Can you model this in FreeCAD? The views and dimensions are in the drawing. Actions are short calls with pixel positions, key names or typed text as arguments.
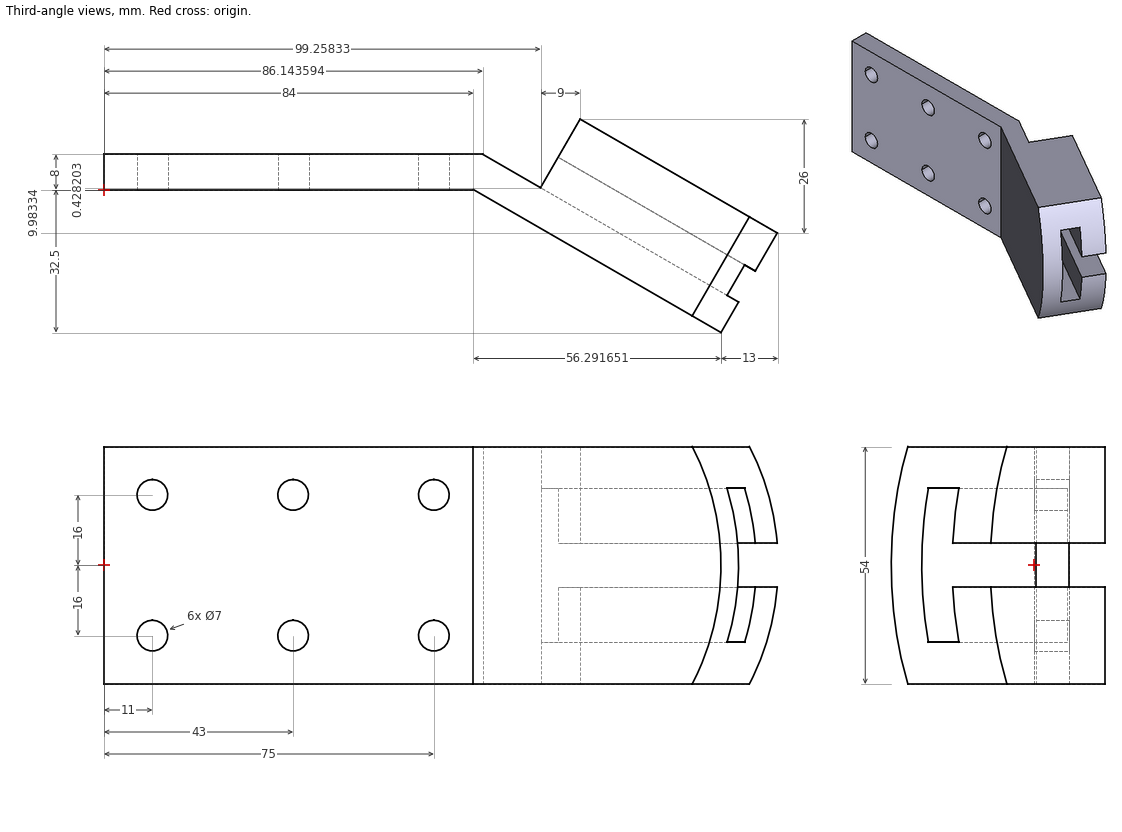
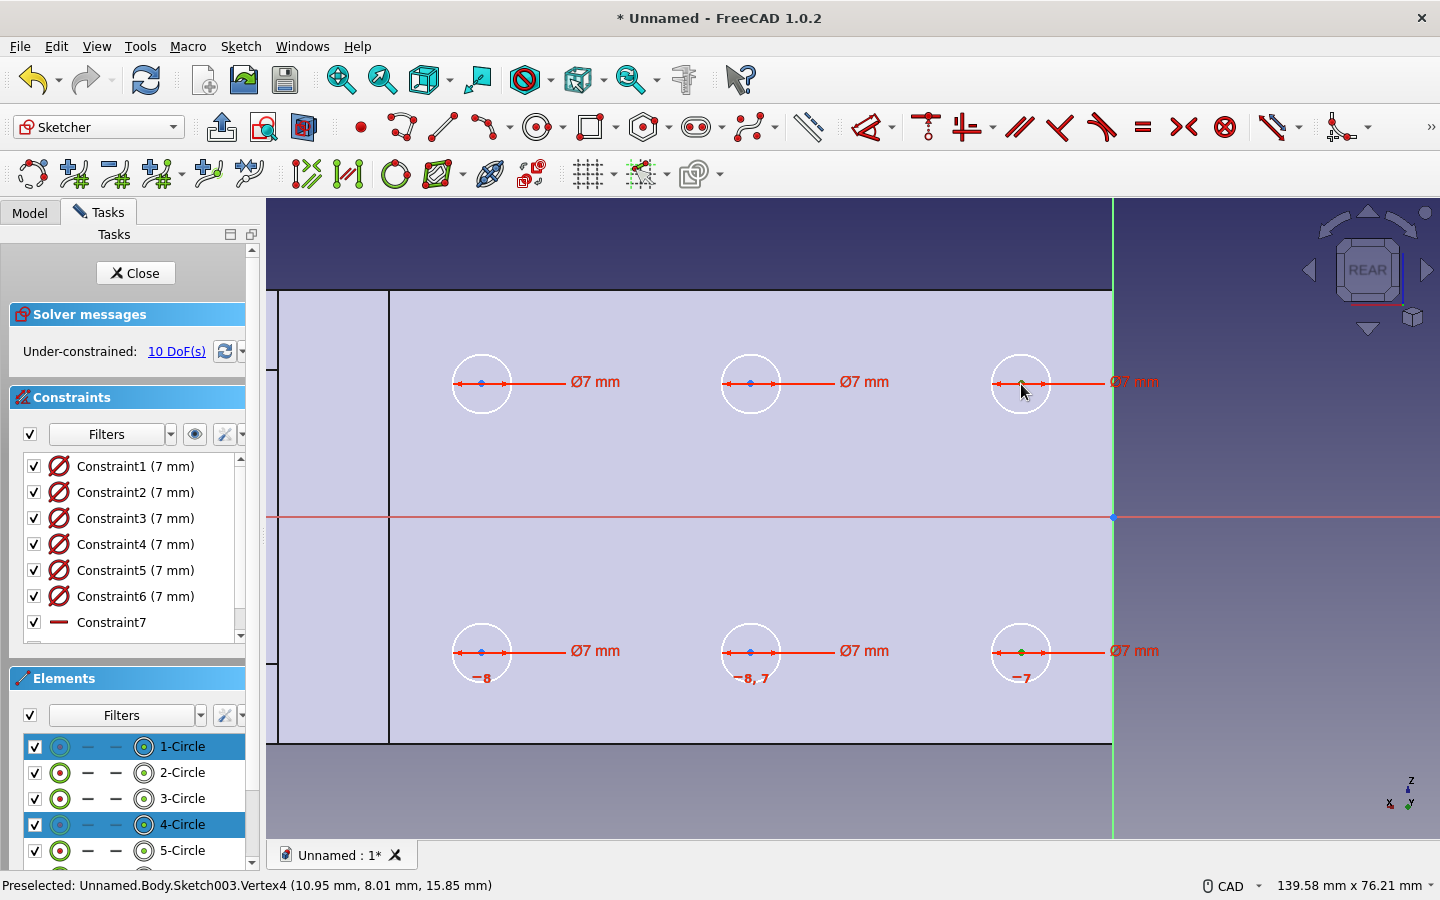
key(v)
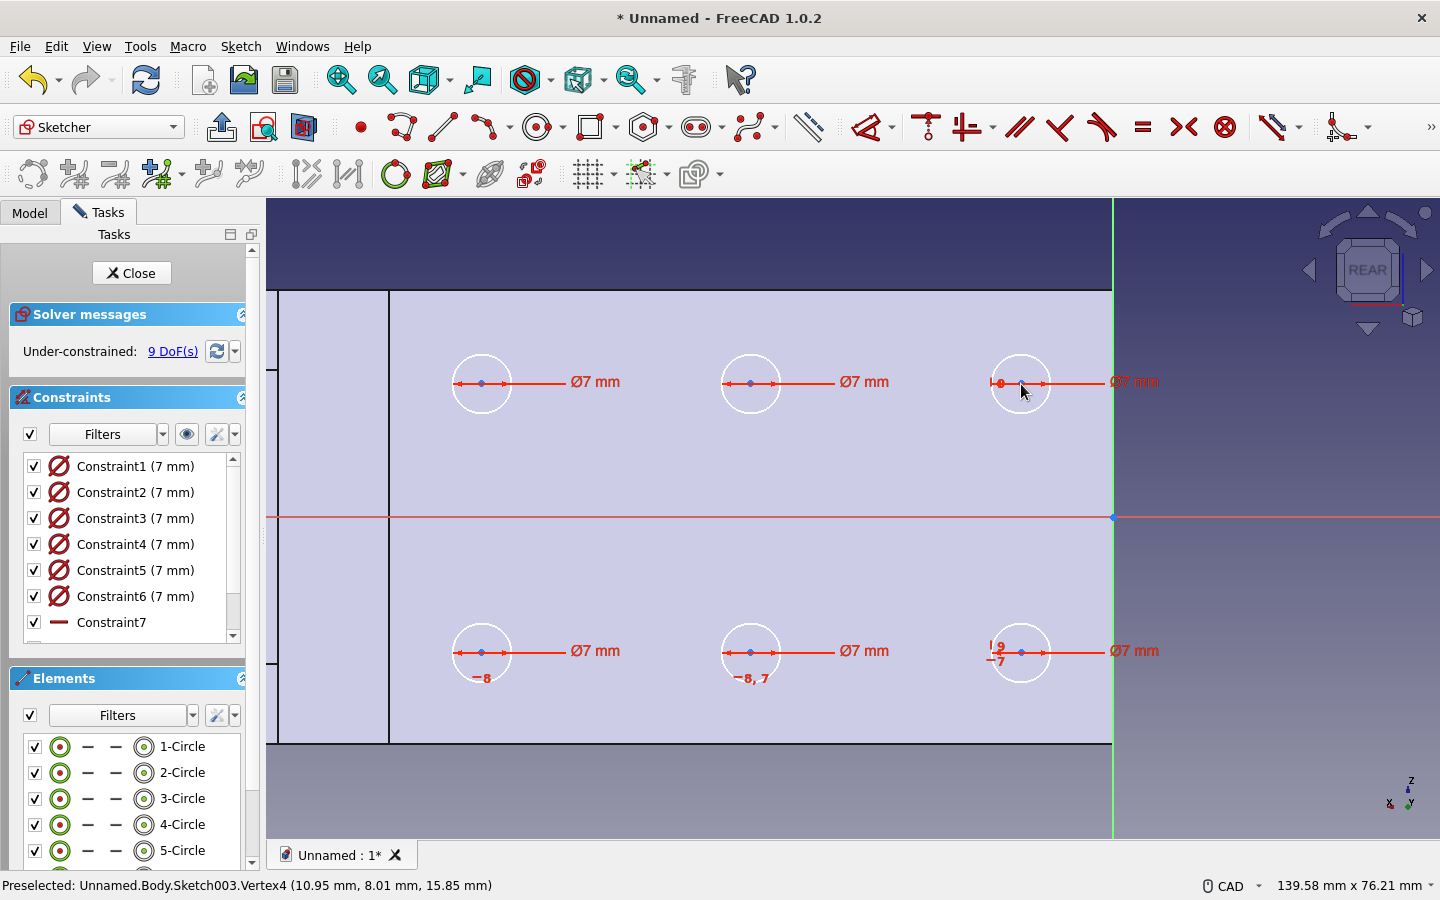
click(751, 653)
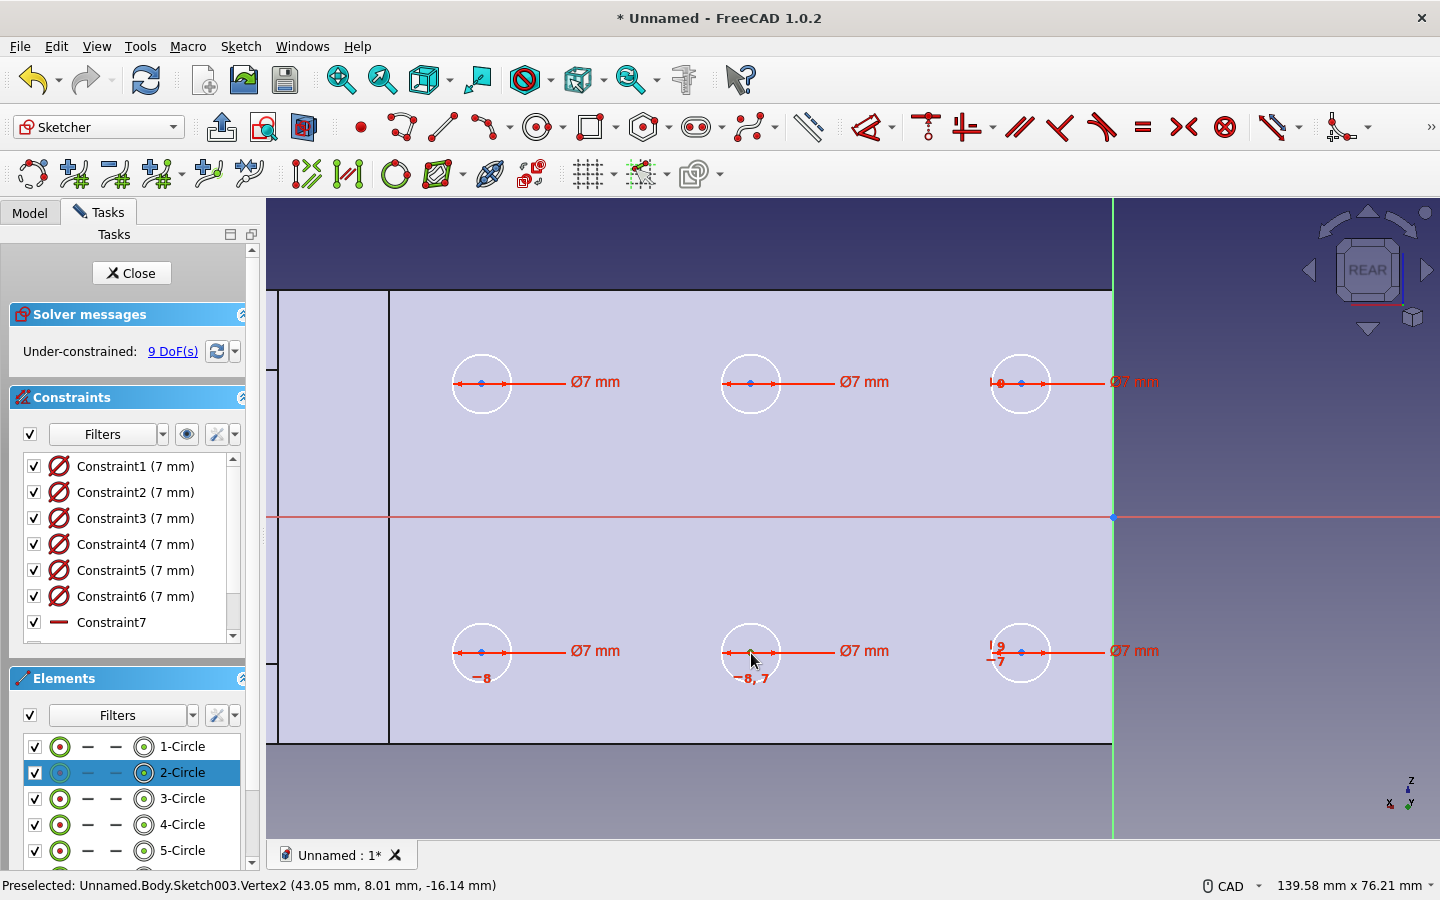
click(751, 384)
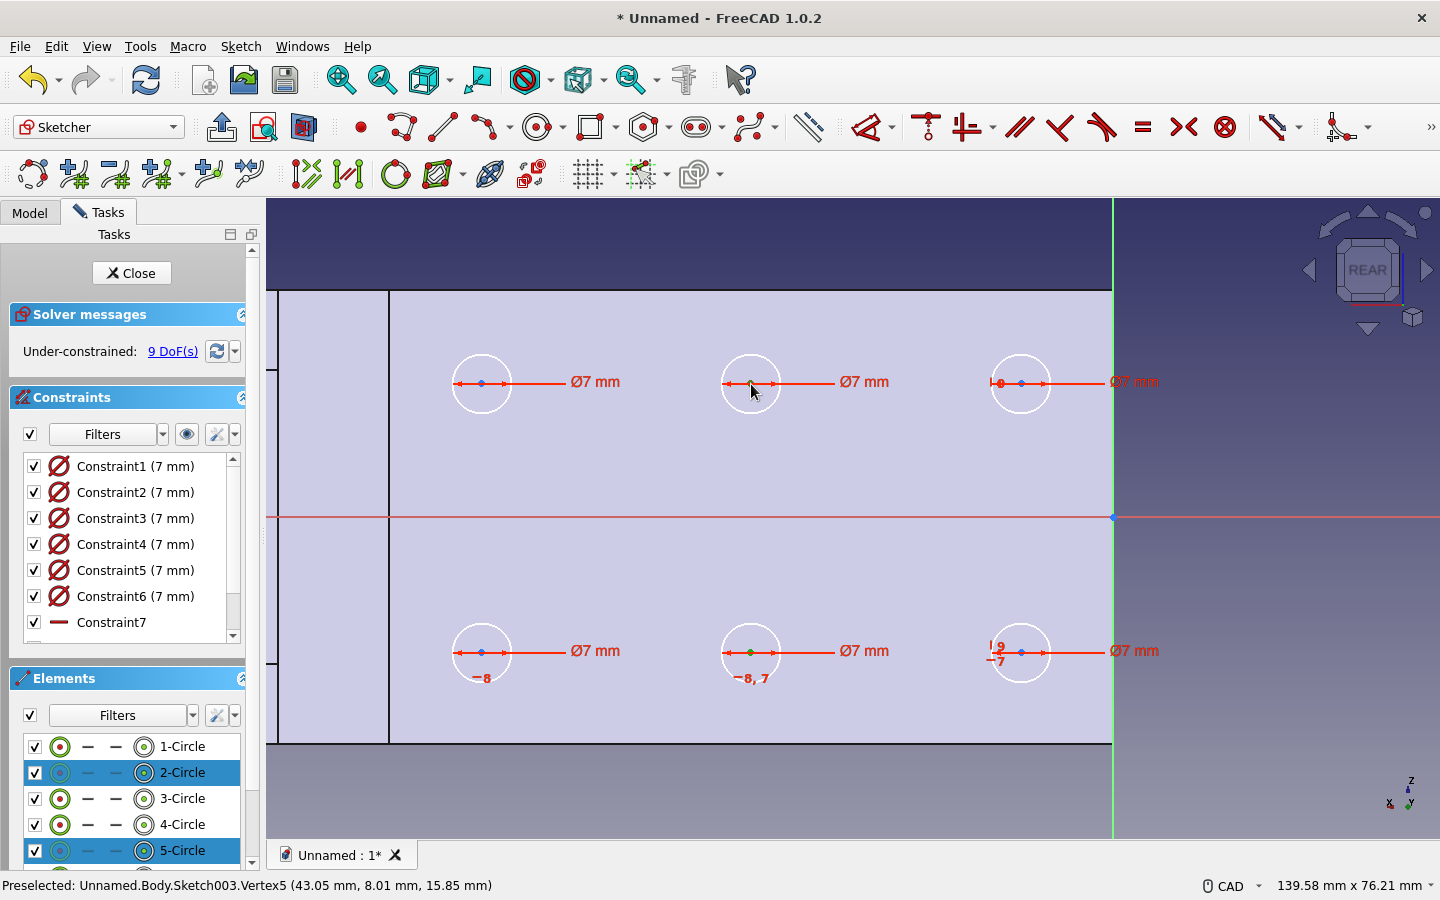
key(v)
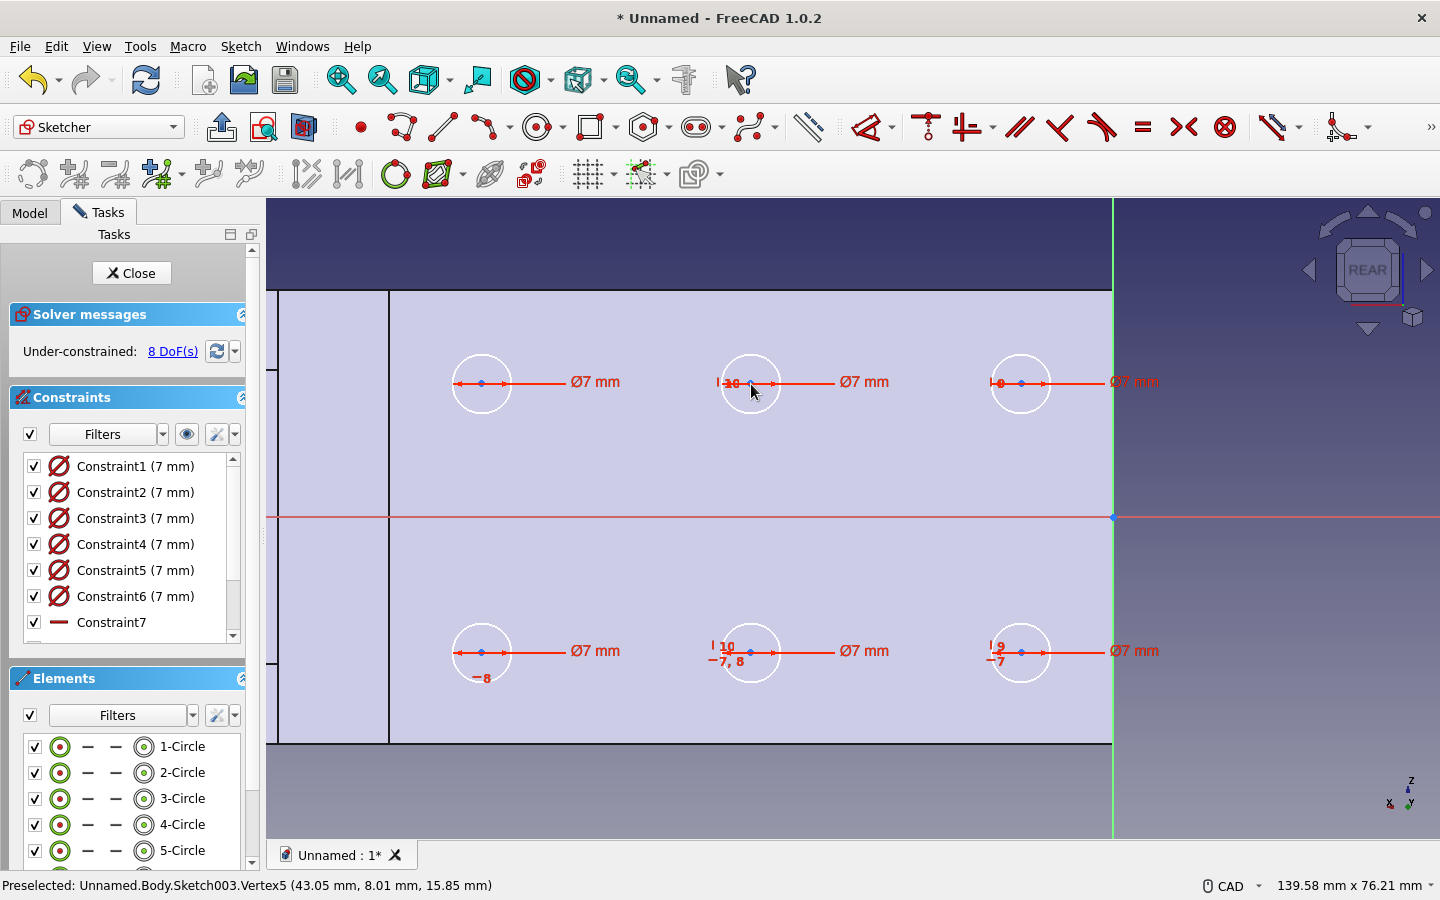
click(1021, 384)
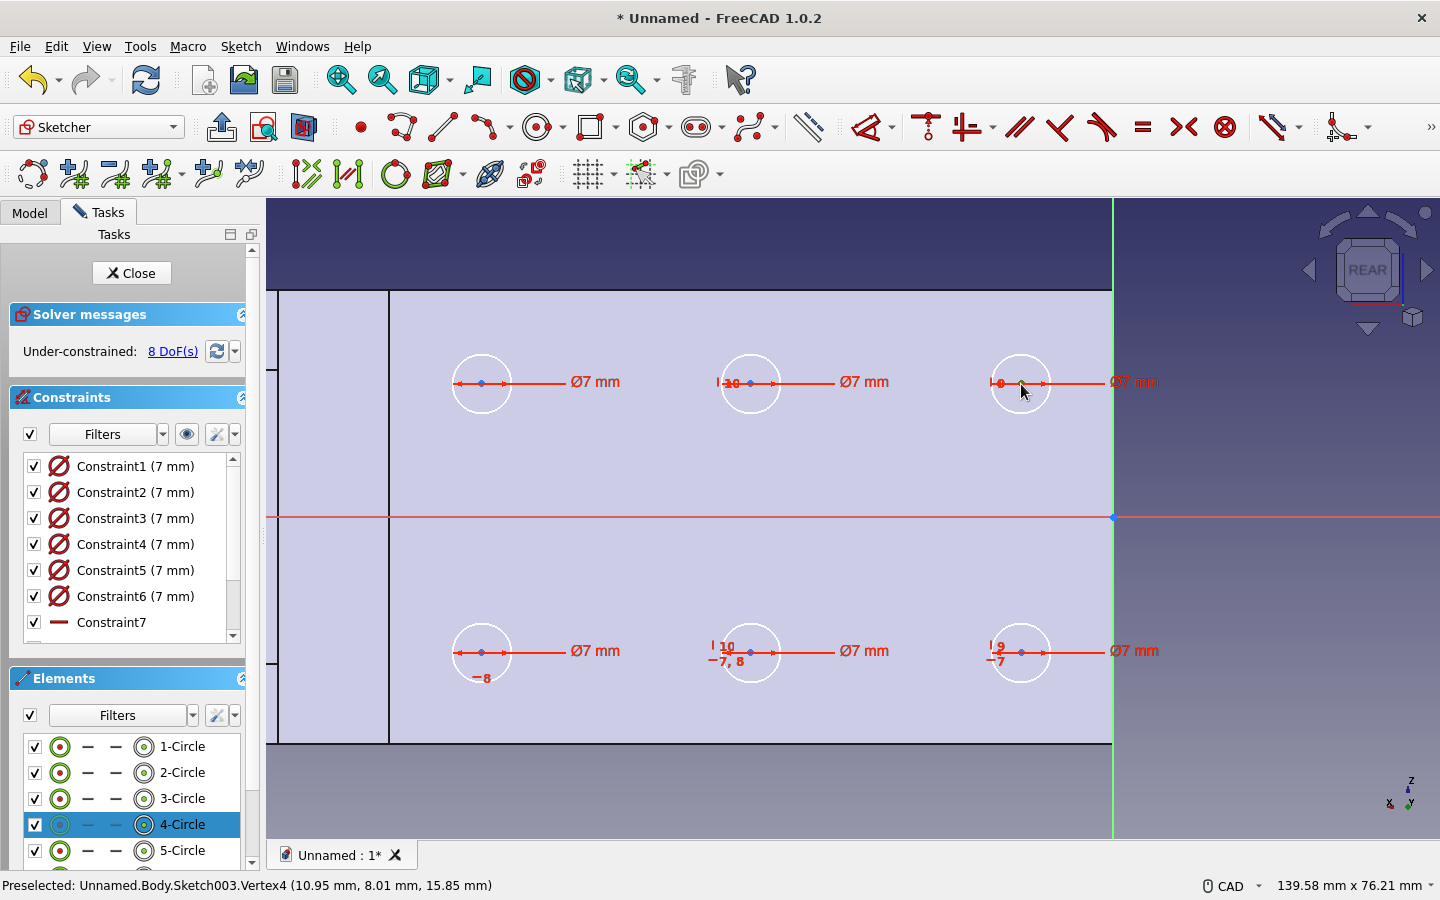
click(751, 384)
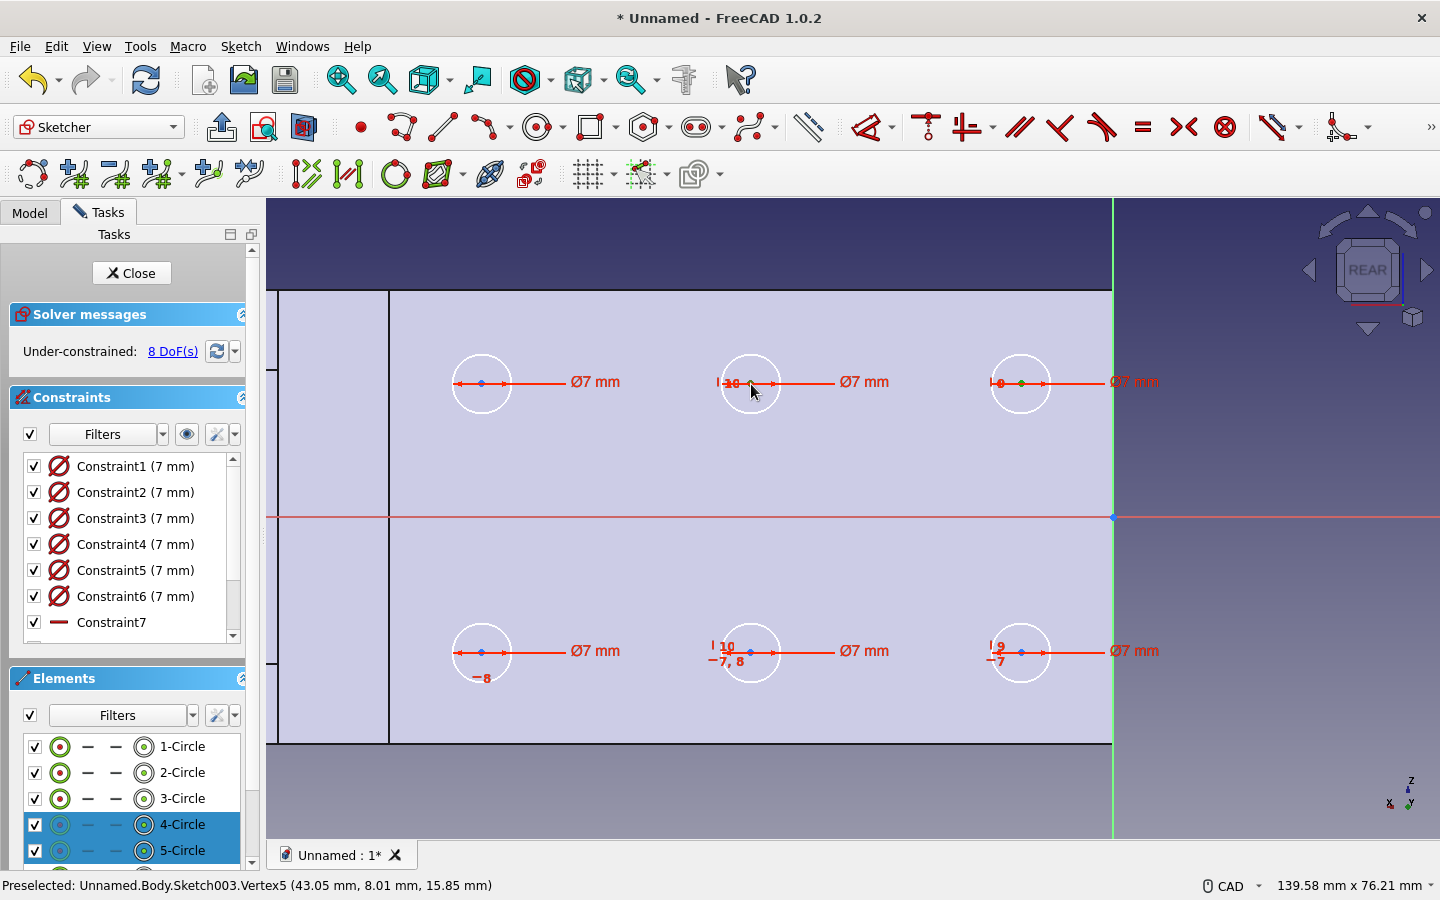
key(h)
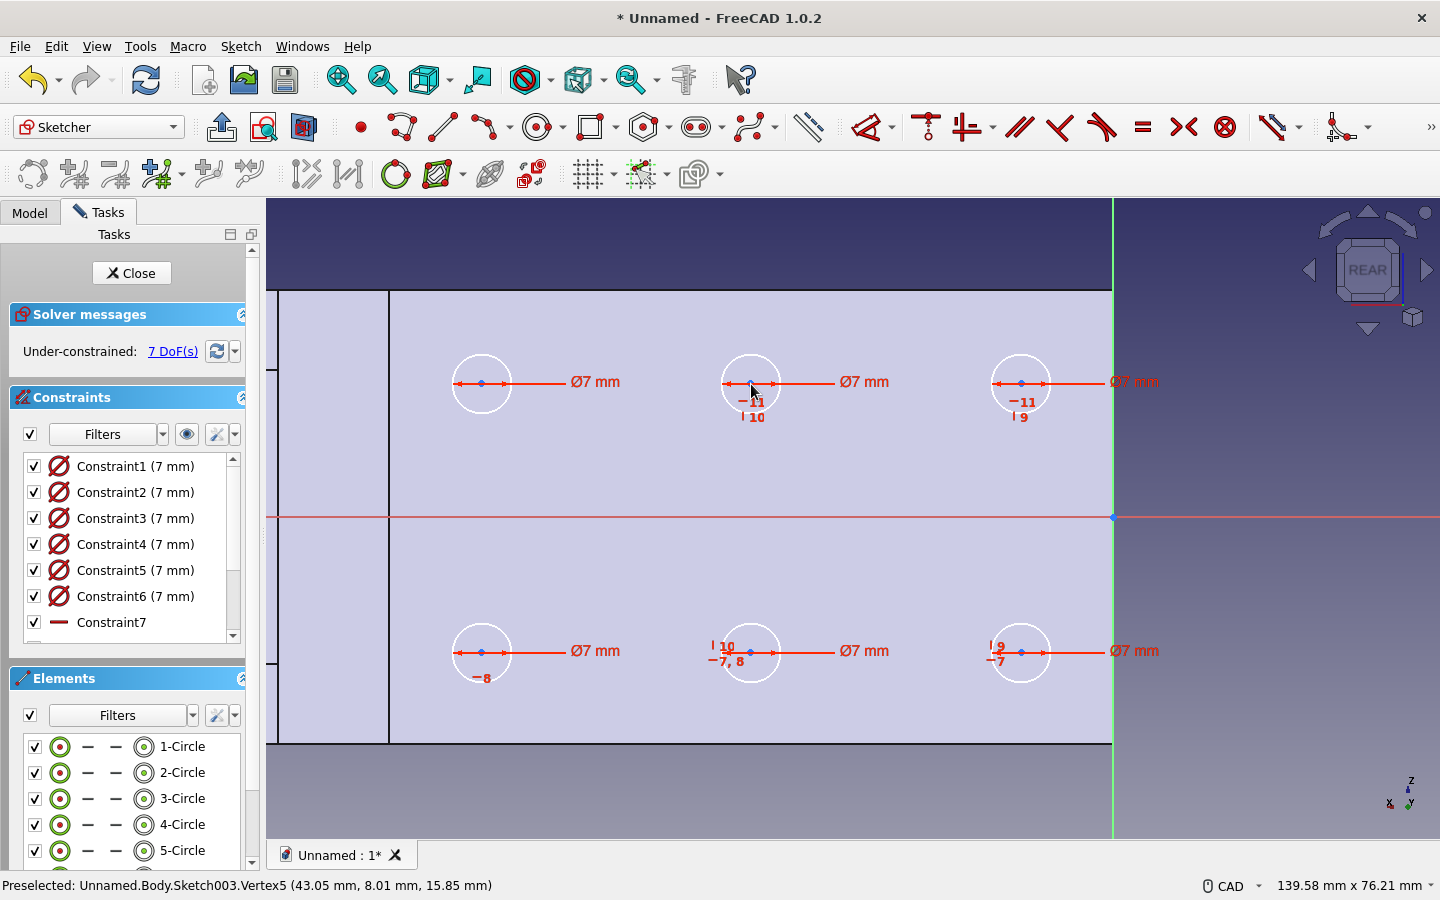
click(482, 653)